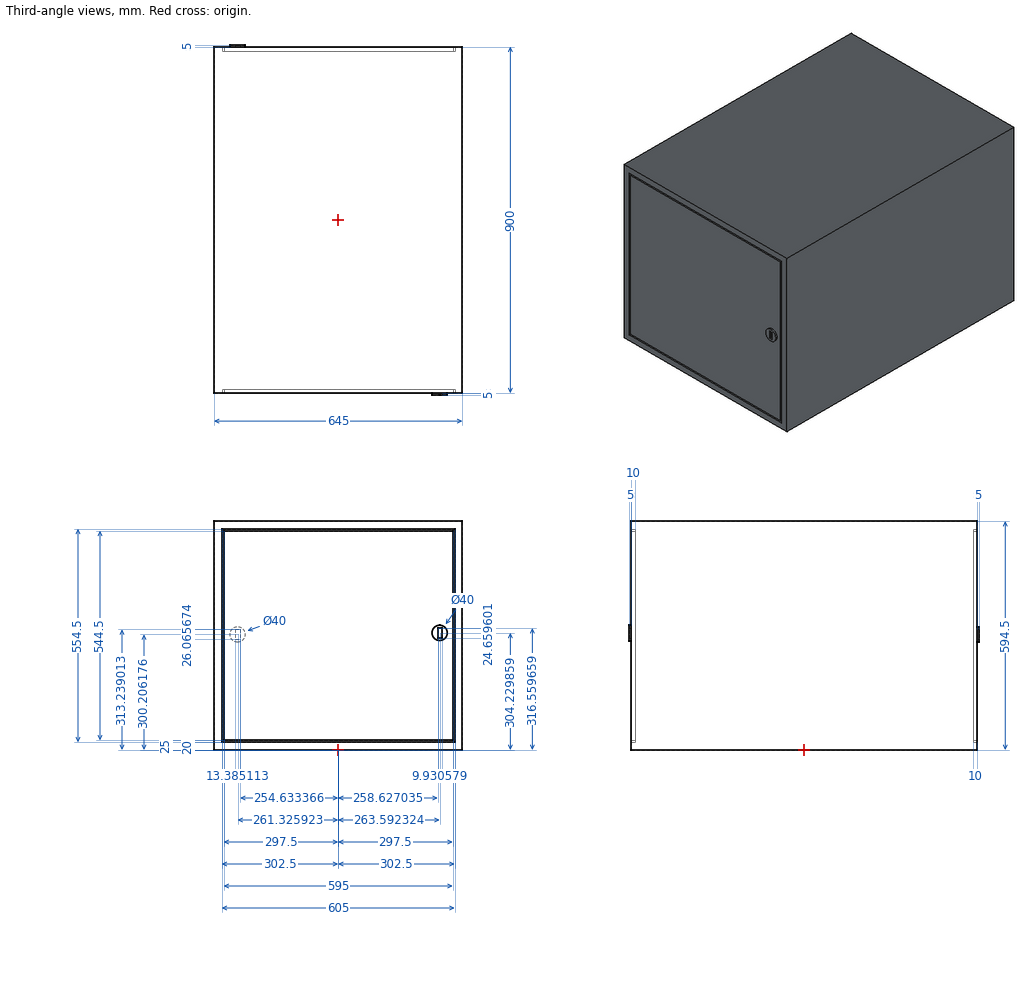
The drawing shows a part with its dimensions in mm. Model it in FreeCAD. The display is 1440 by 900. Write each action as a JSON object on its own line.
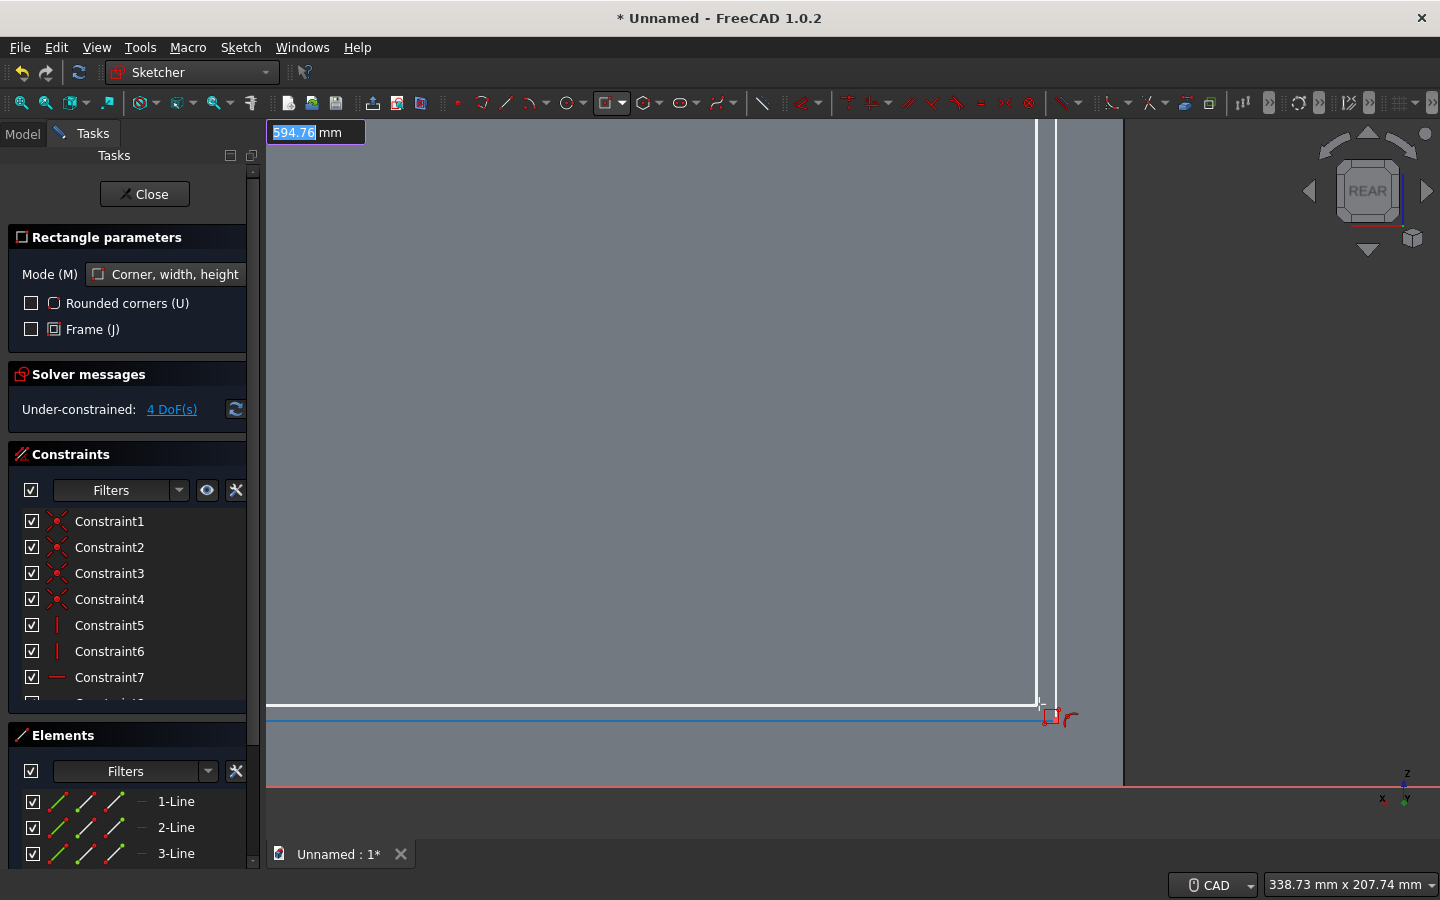
{"action": "left_click", "coordinate": [1037, 700]}
{"action": "key", "text": "Escape"}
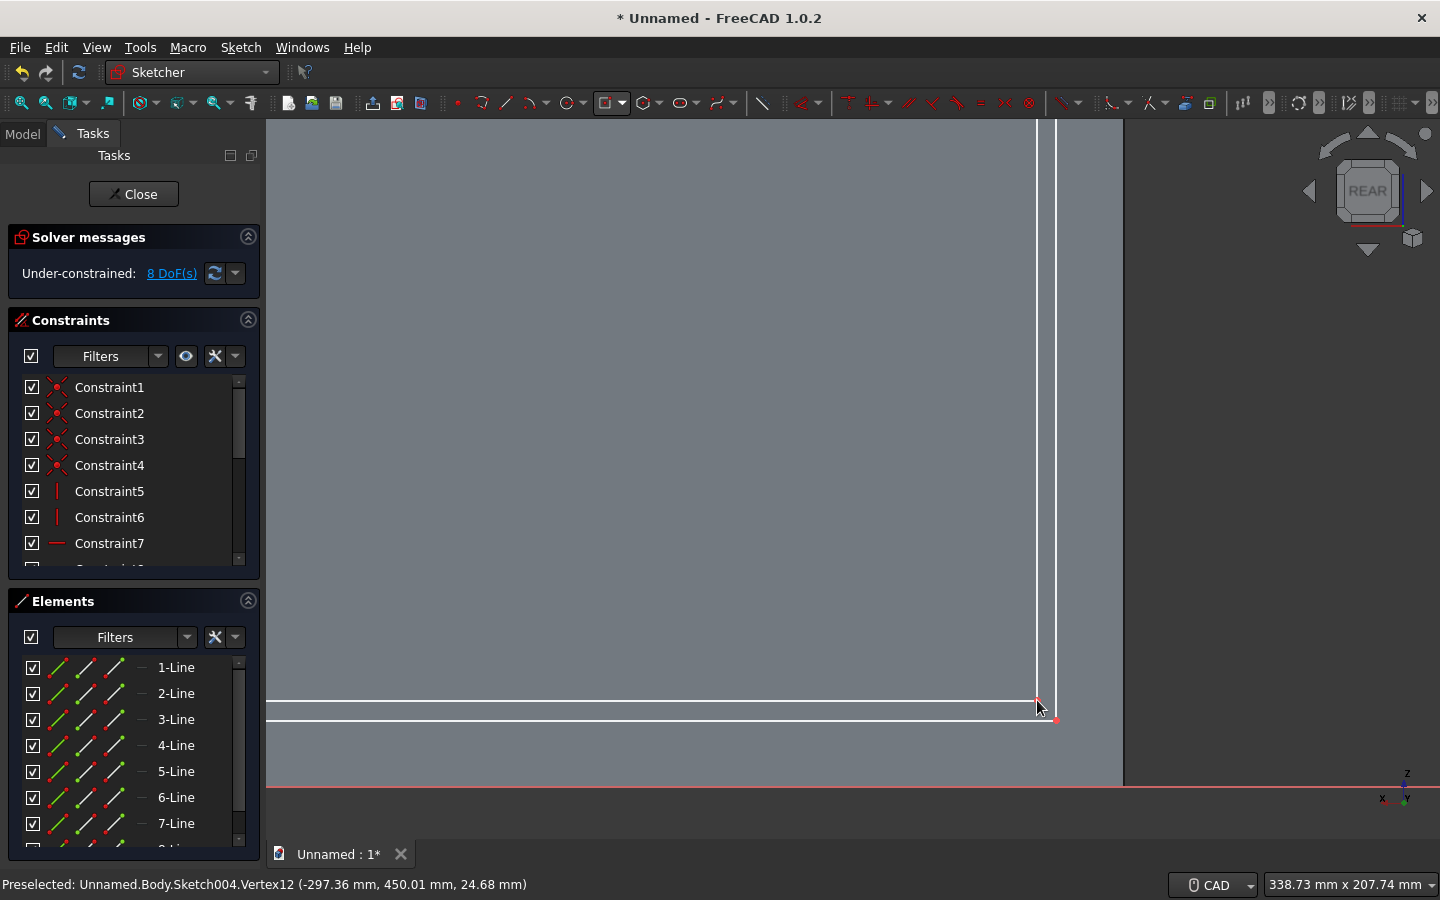
{"action": "key", "text": "d"}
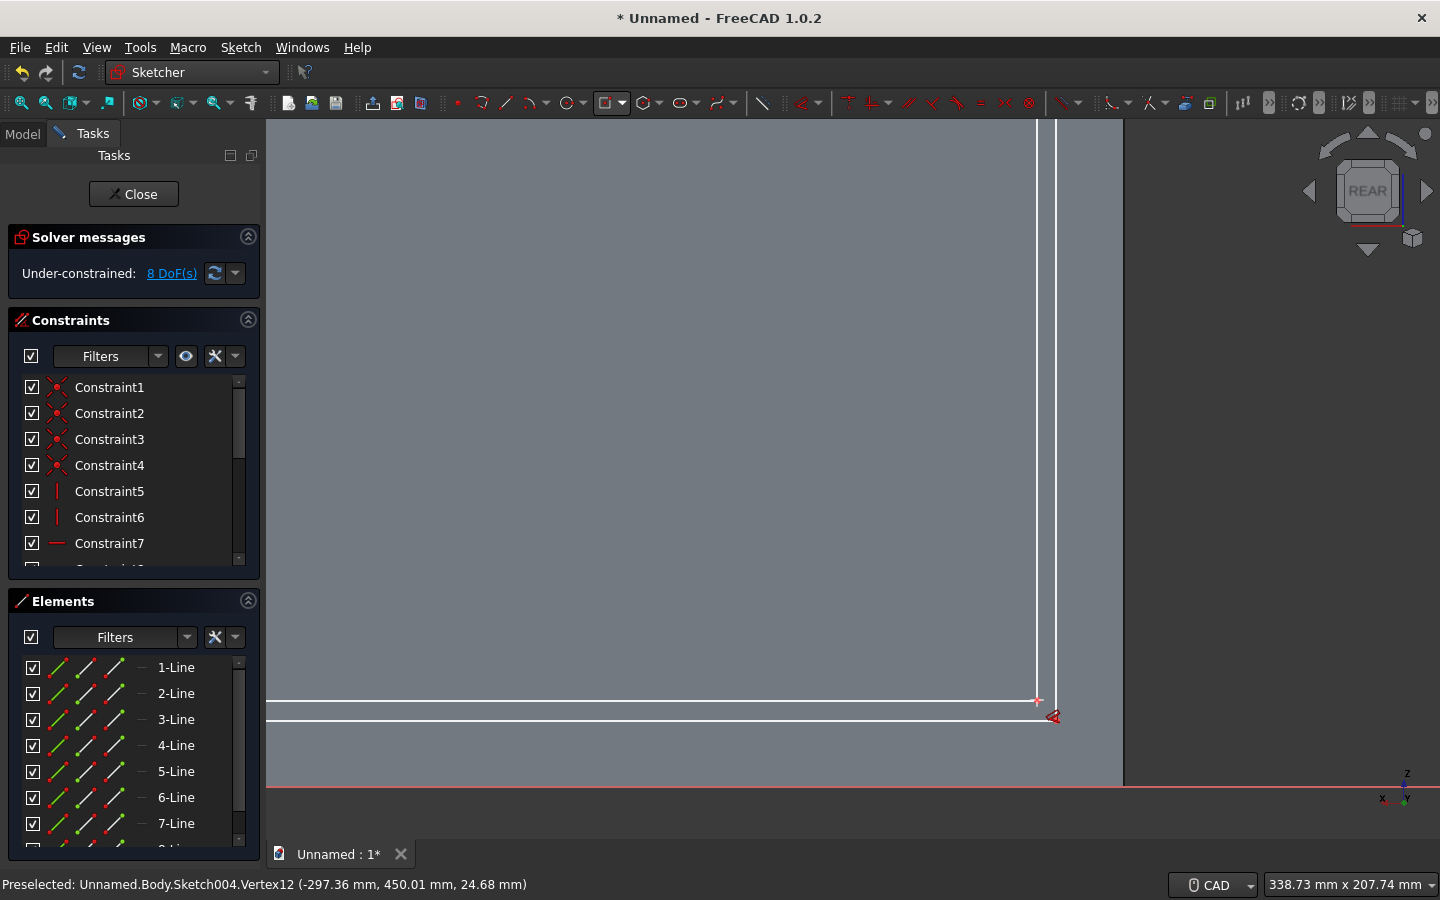
{"action": "left_click", "coordinate": [427, 721]}
{"action": "left_click", "coordinate": [675, 755]}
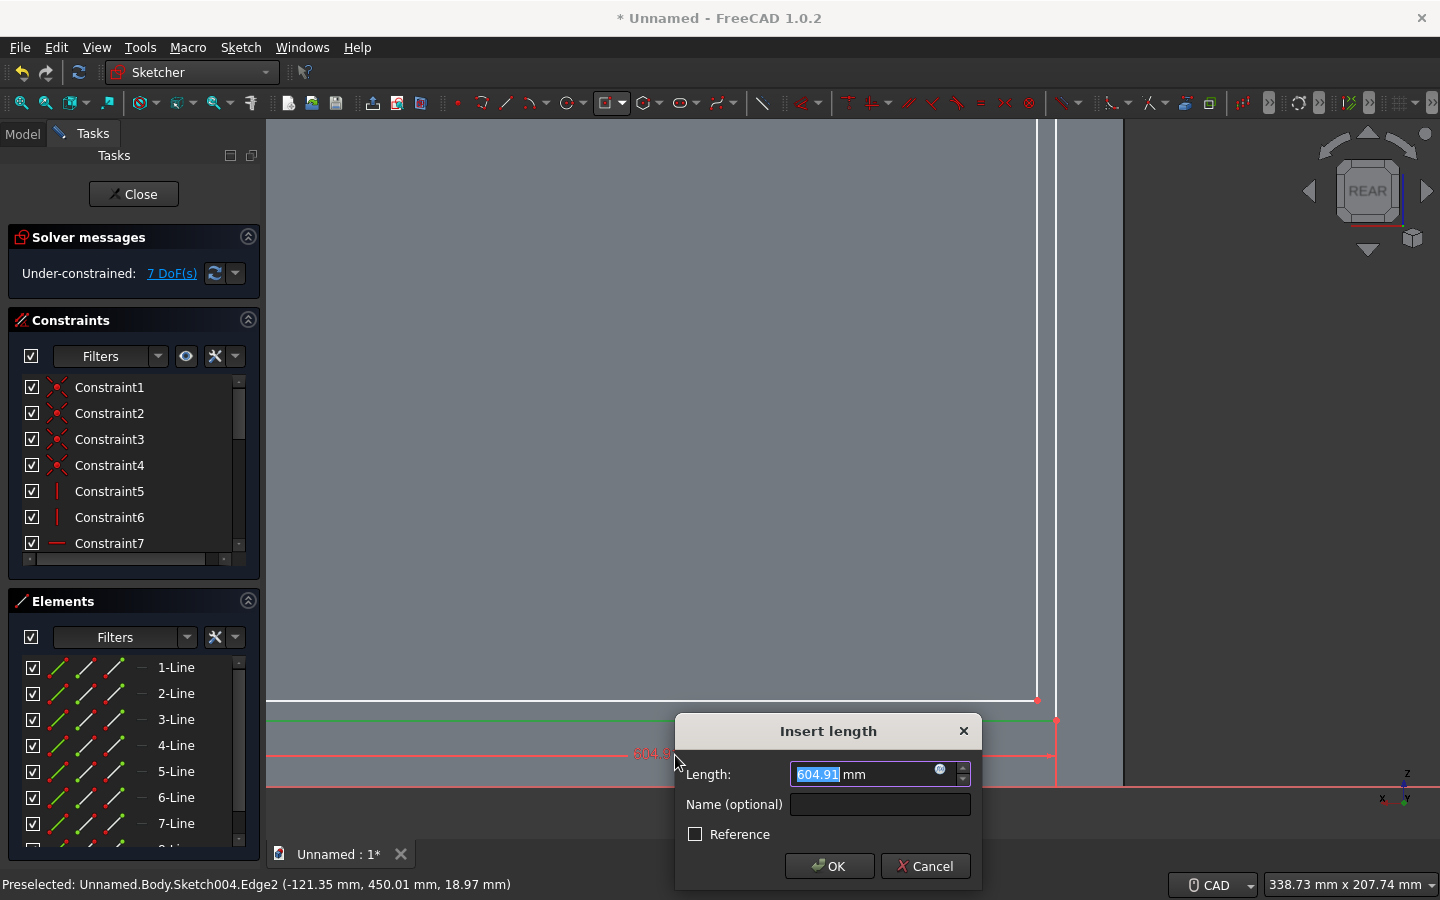
{"action": "type", "text": "605"}
{"action": "key", "text": "Return"}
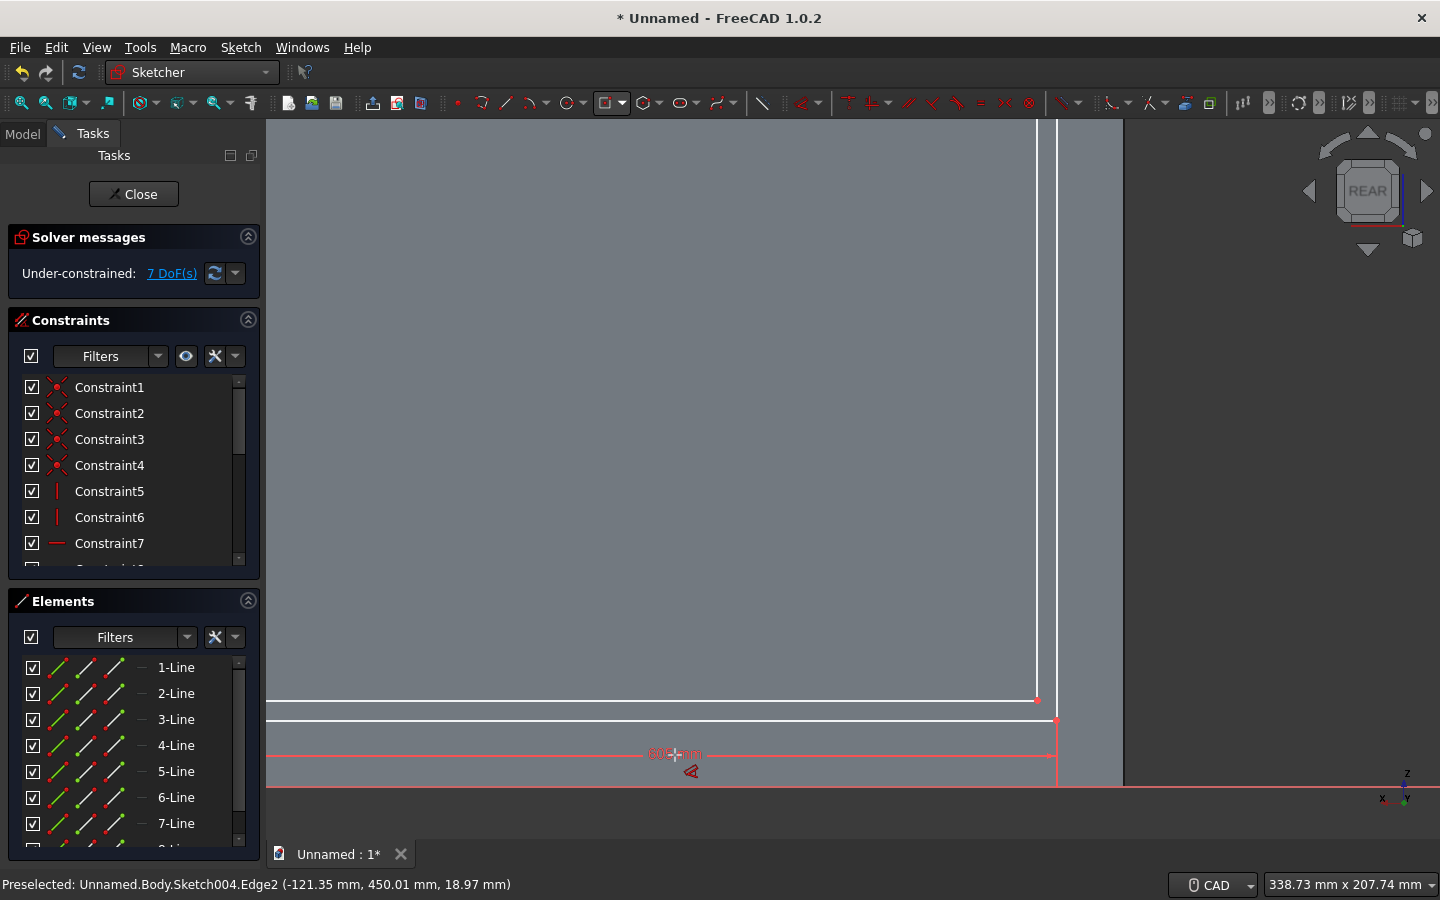
{"action": "left_click", "coordinate": [419, 701]}
{"action": "left_click", "coordinate": [495, 735]}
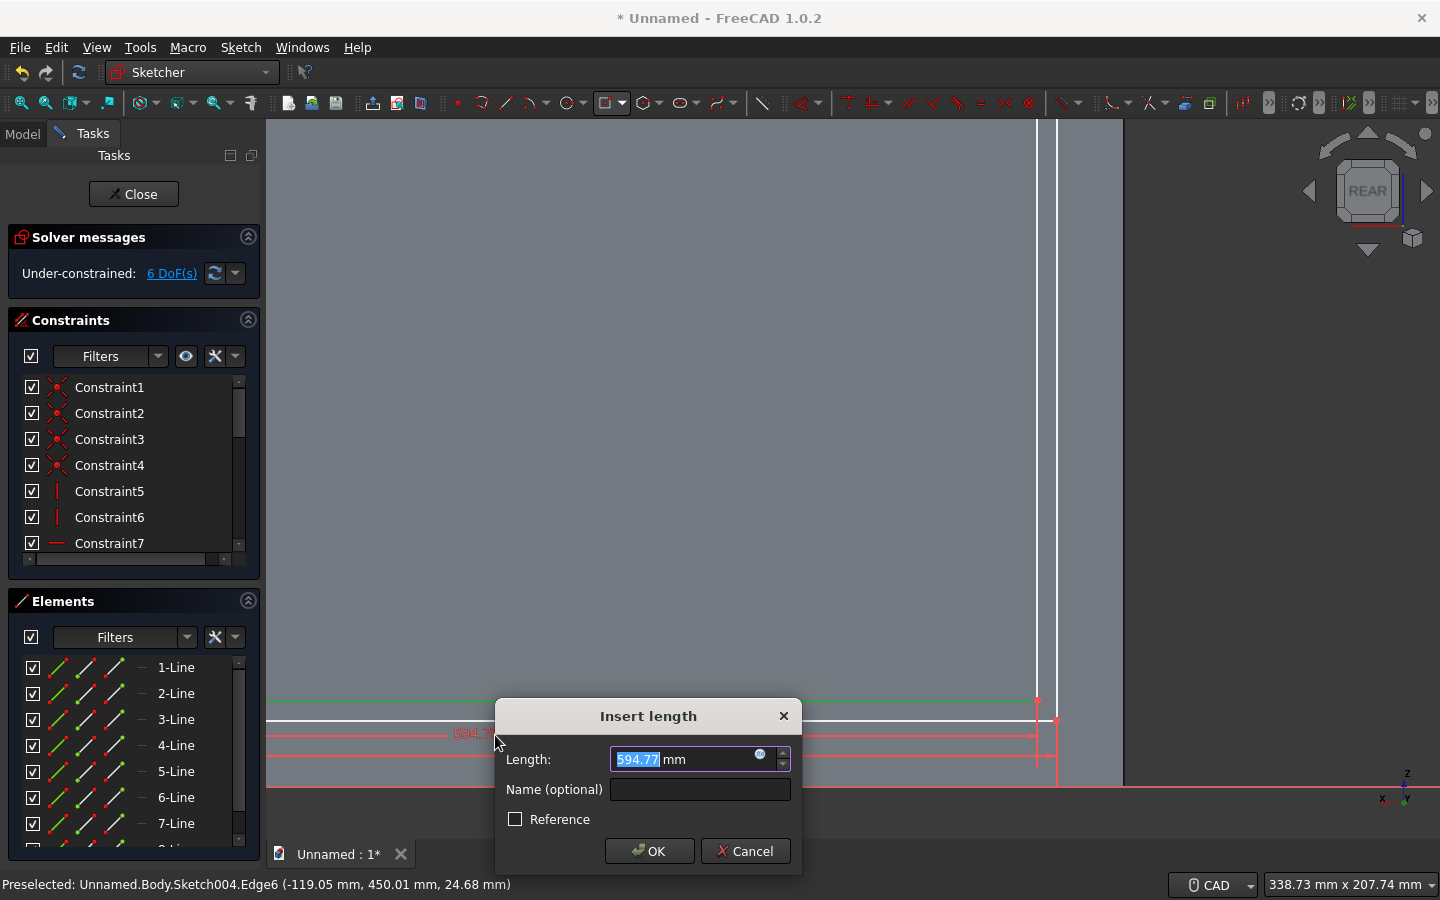
{"action": "type", "text": "595"}
{"action": "key", "text": "Return"}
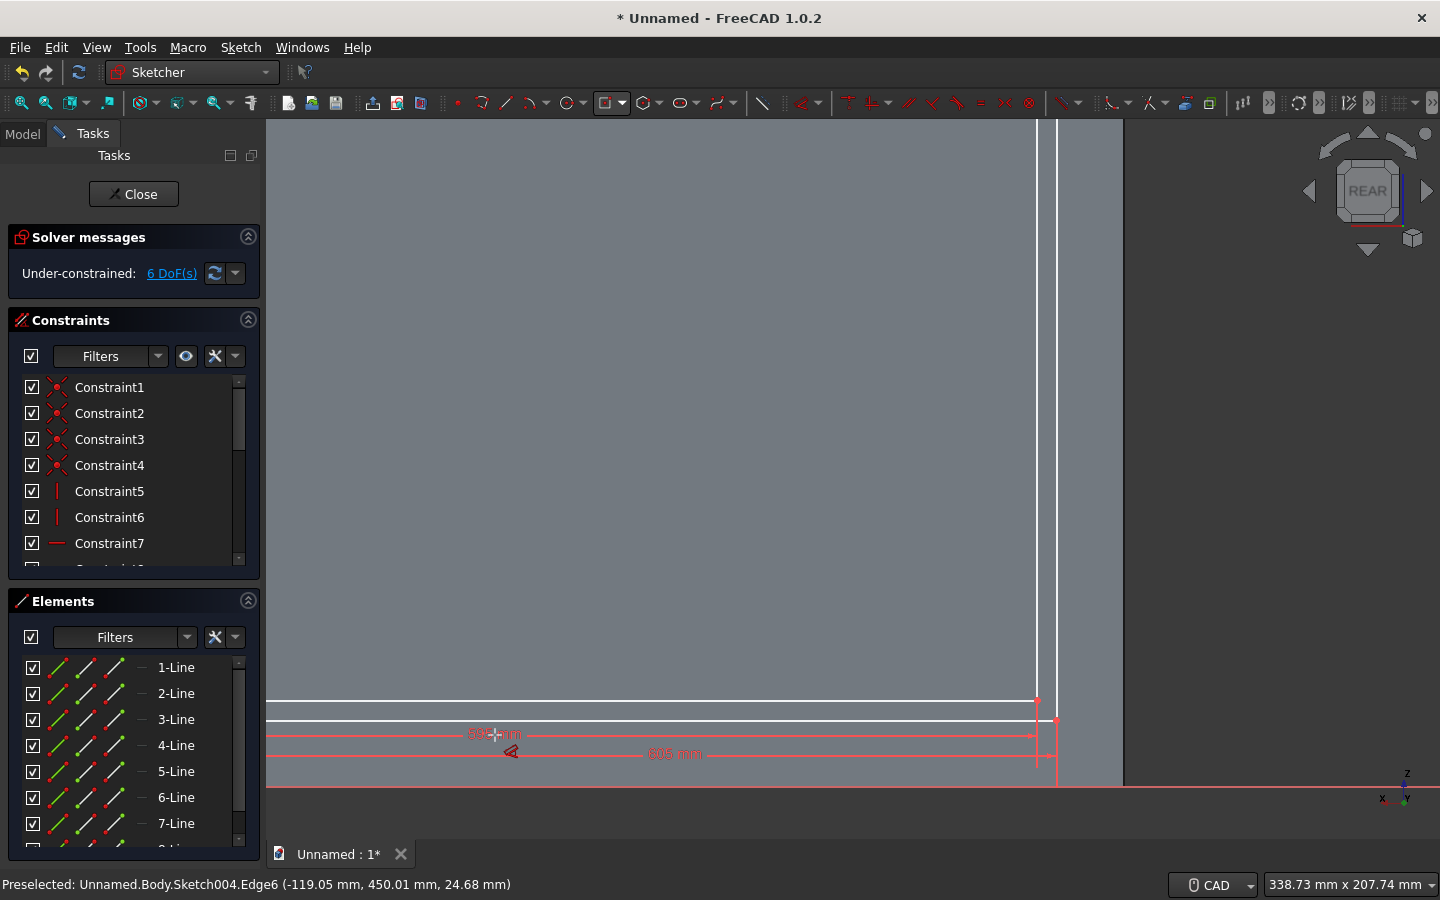
{"action": "scroll", "coordinate": [1039, 704], "scroll_direction": "down", "scroll_amount": 7}